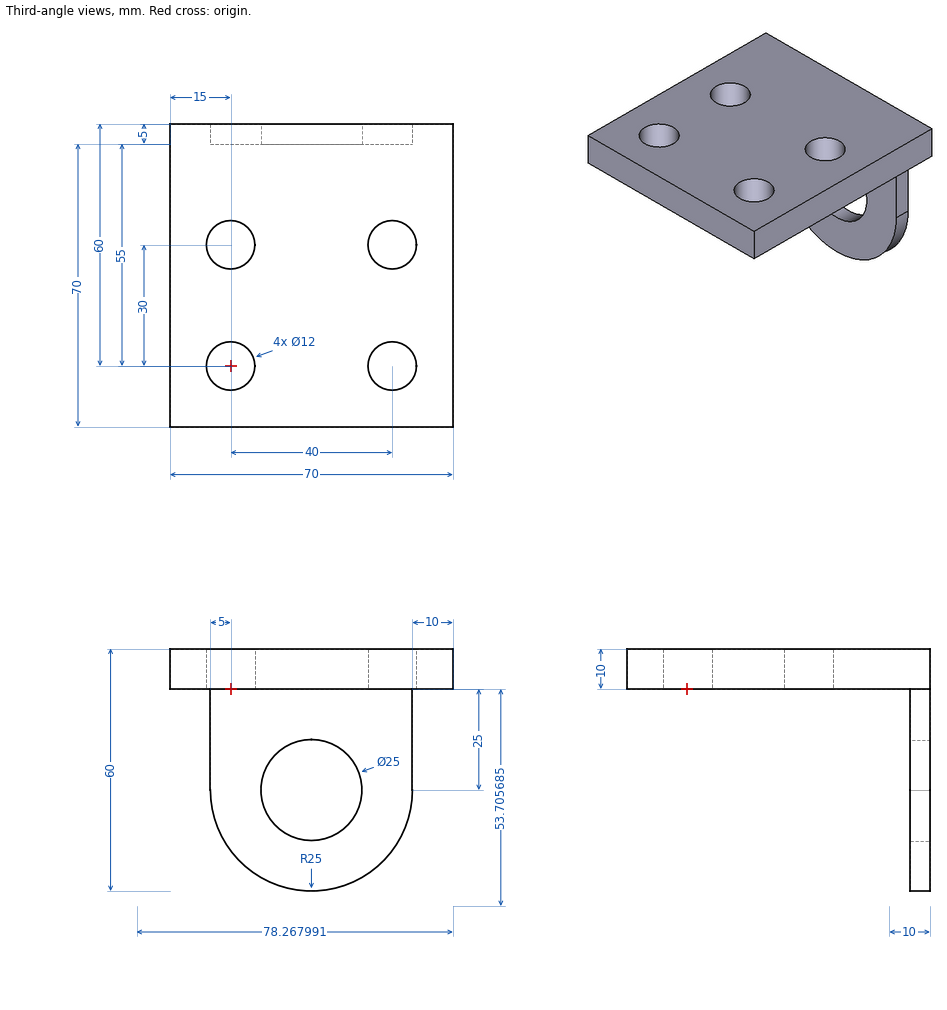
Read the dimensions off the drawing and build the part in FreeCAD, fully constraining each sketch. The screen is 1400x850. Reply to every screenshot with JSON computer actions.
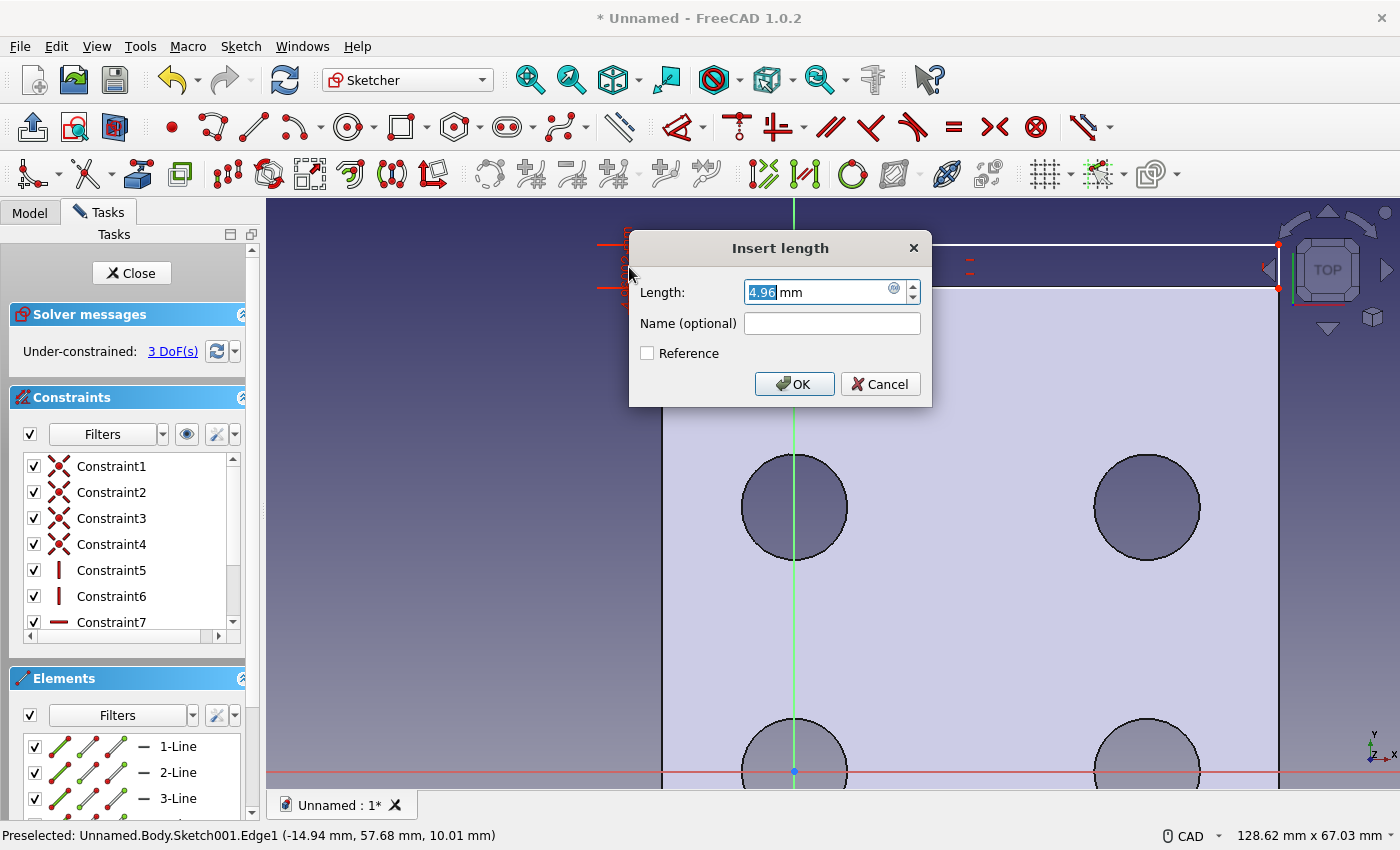
{"action": "type", "text": "5"}
{"action": "key", "text": "Return"}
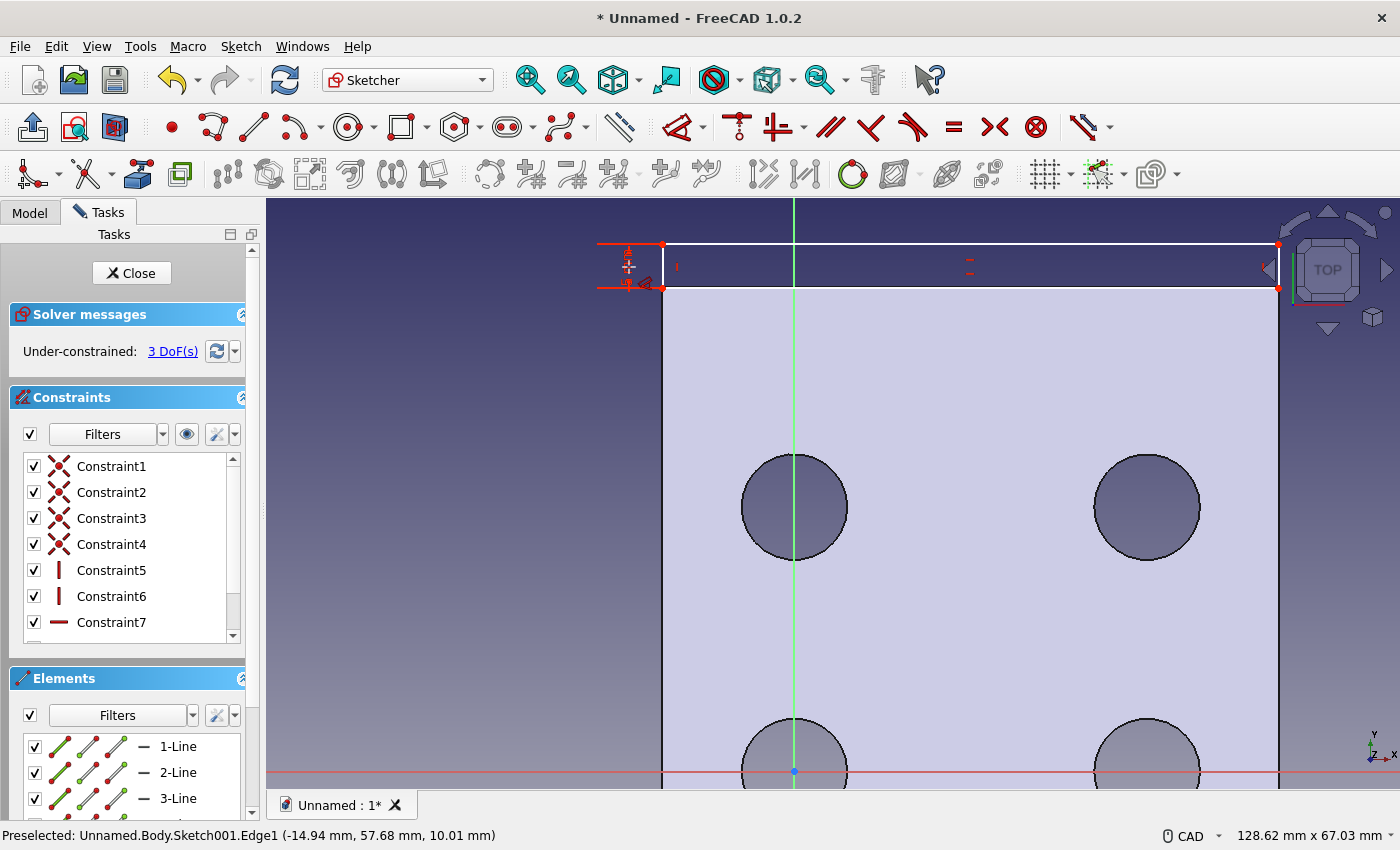
{"action": "left_click", "coordinate": [847, 288]}
{"action": "left_click", "coordinate": [949, 322]}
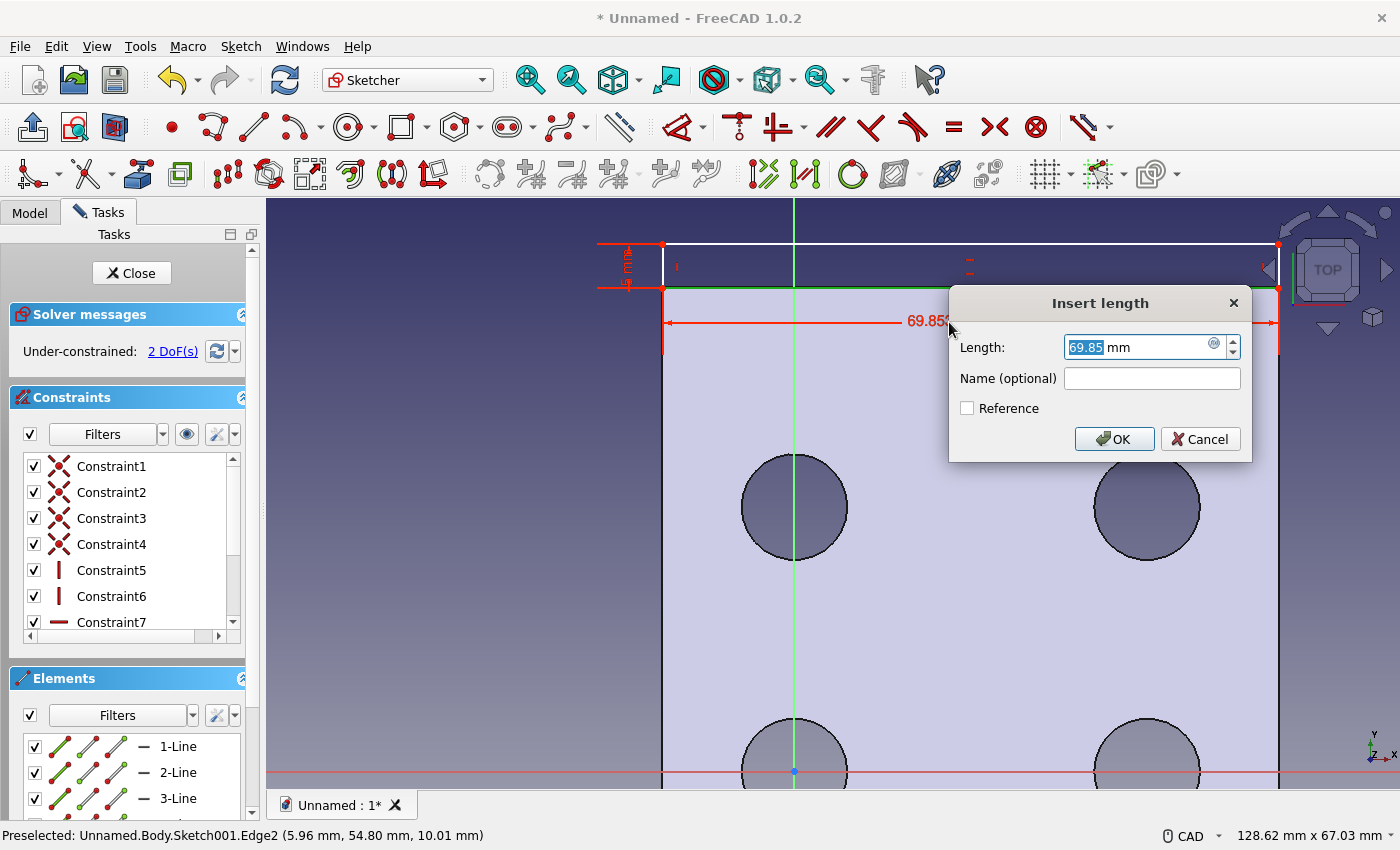
{"action": "type", "text": "70"}
{"action": "key", "text": "Return"}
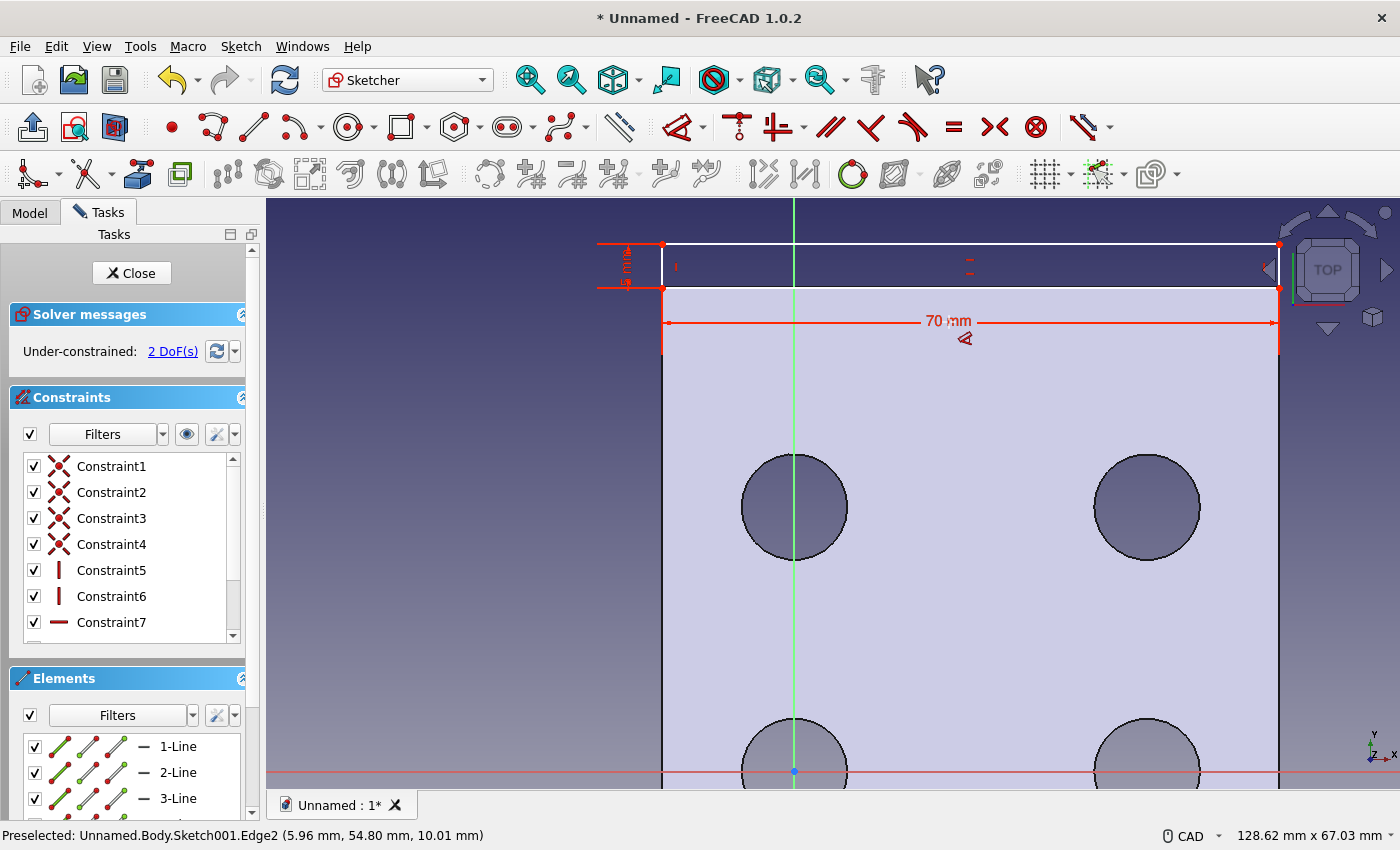
{"action": "left_click", "coordinate": [662, 244]}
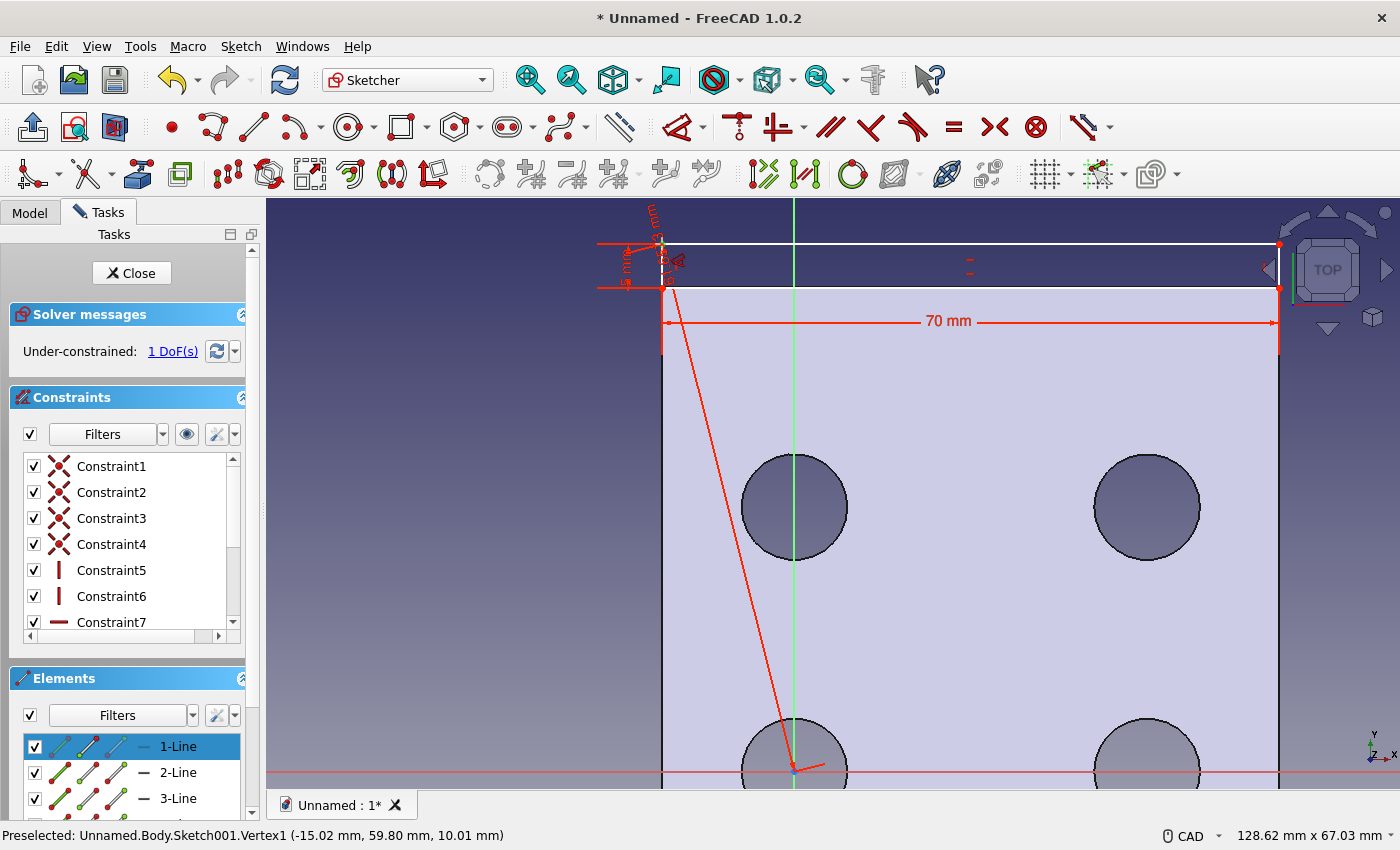
{"action": "key", "text": "Escape"}
{"action": "key", "text": "Escape"}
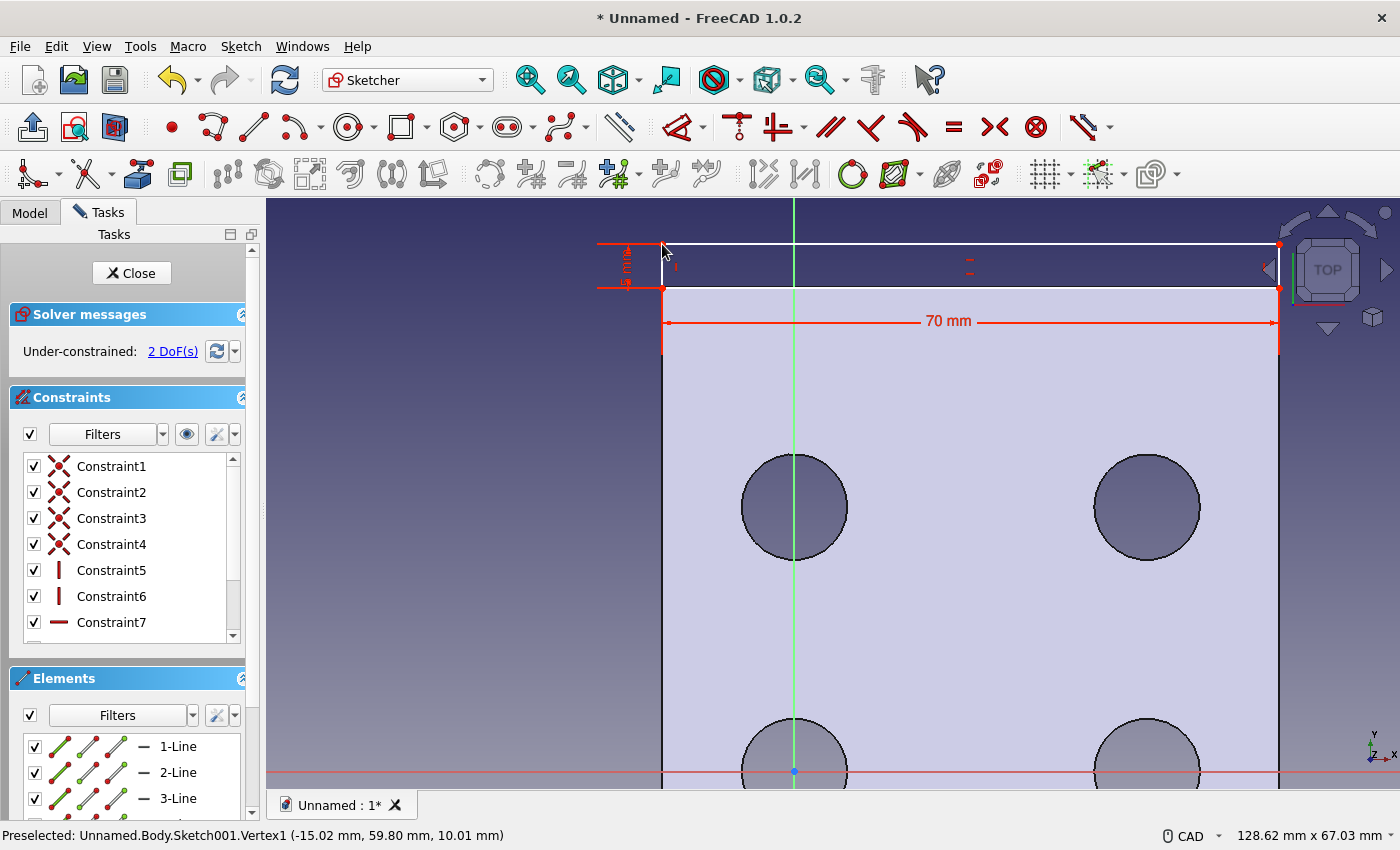
{"action": "left_click", "coordinate": [662, 244]}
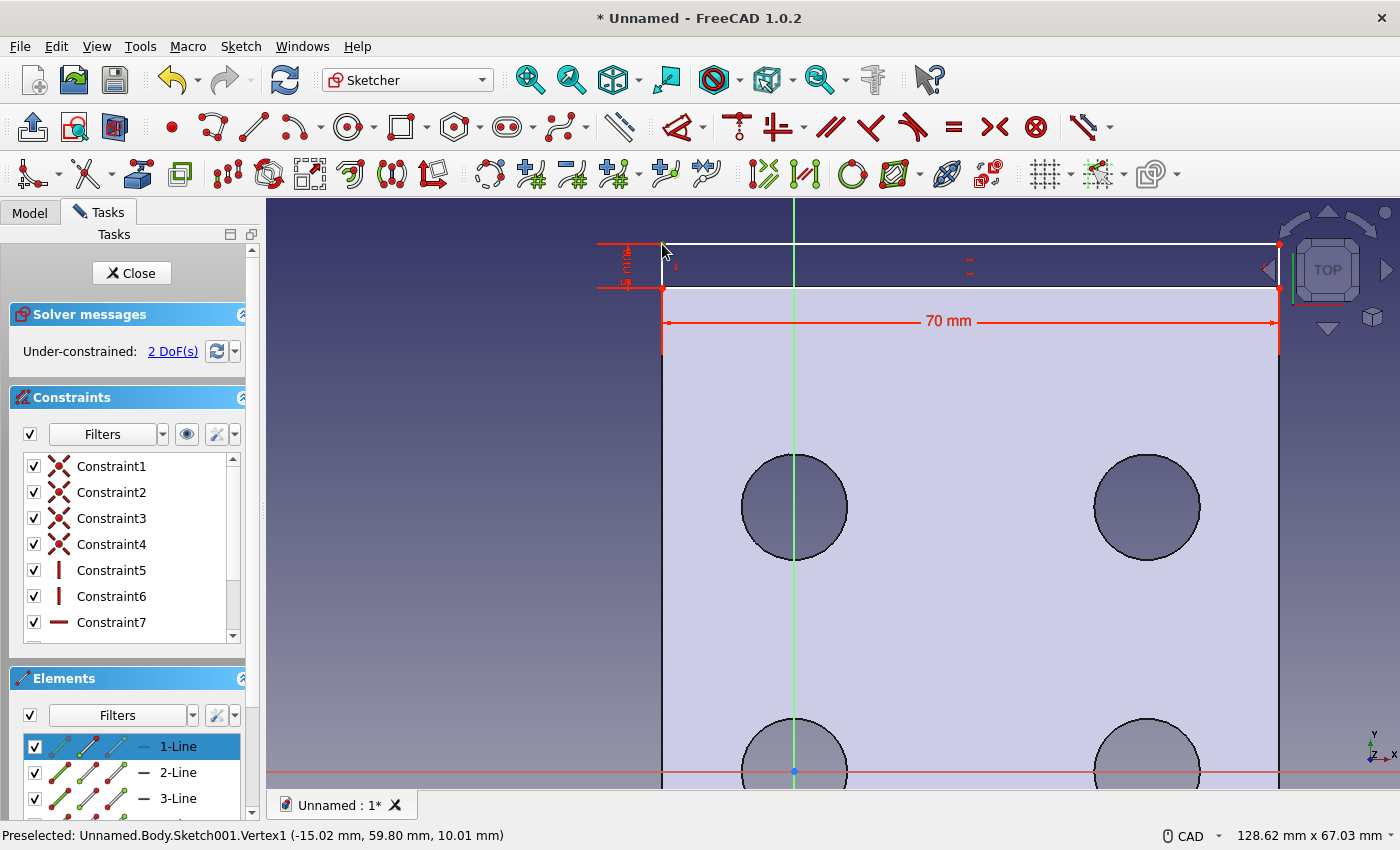
{"action": "key", "text": "l"}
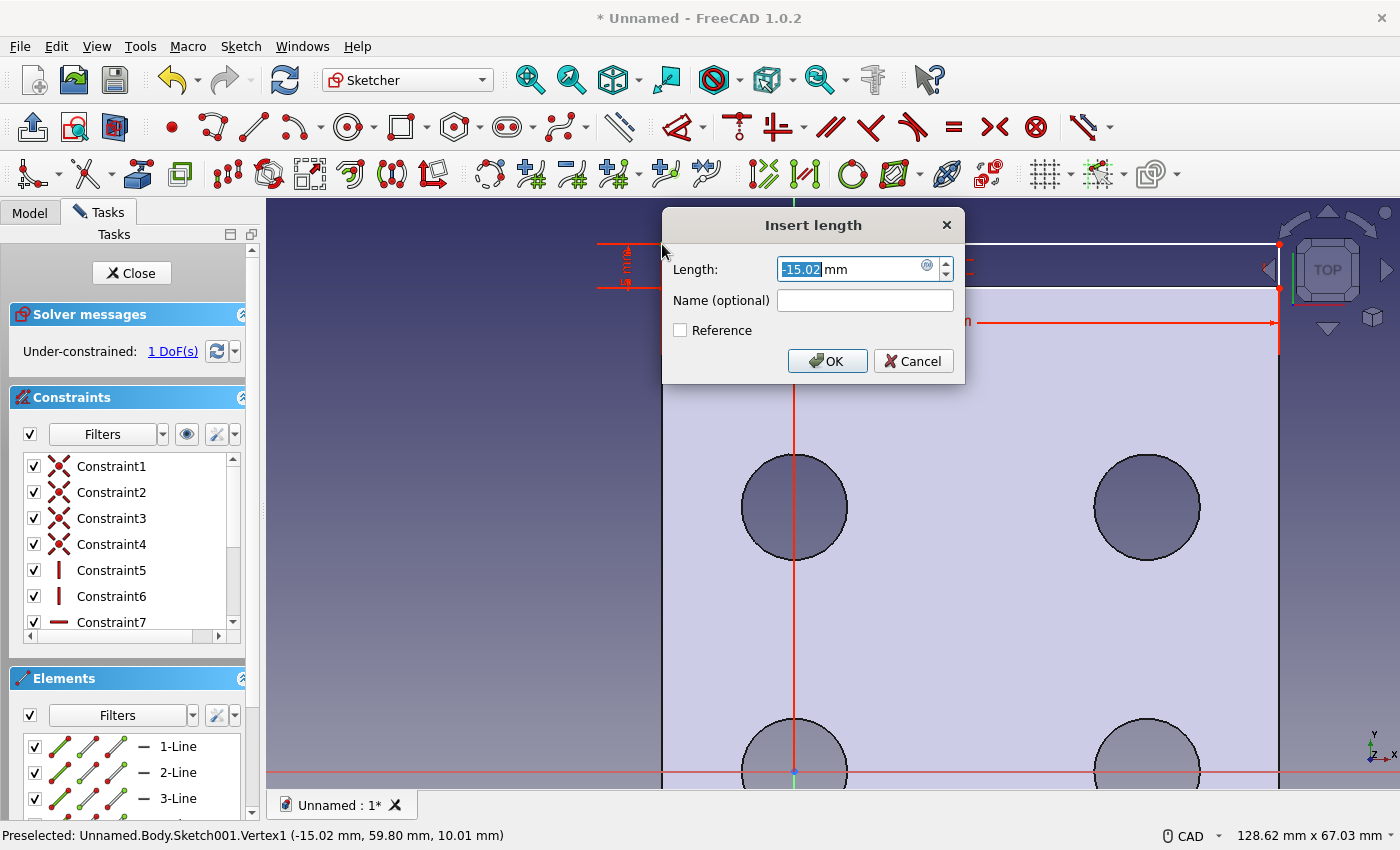
{"action": "type", "text": "-15"}
{"action": "key", "text": "Return"}